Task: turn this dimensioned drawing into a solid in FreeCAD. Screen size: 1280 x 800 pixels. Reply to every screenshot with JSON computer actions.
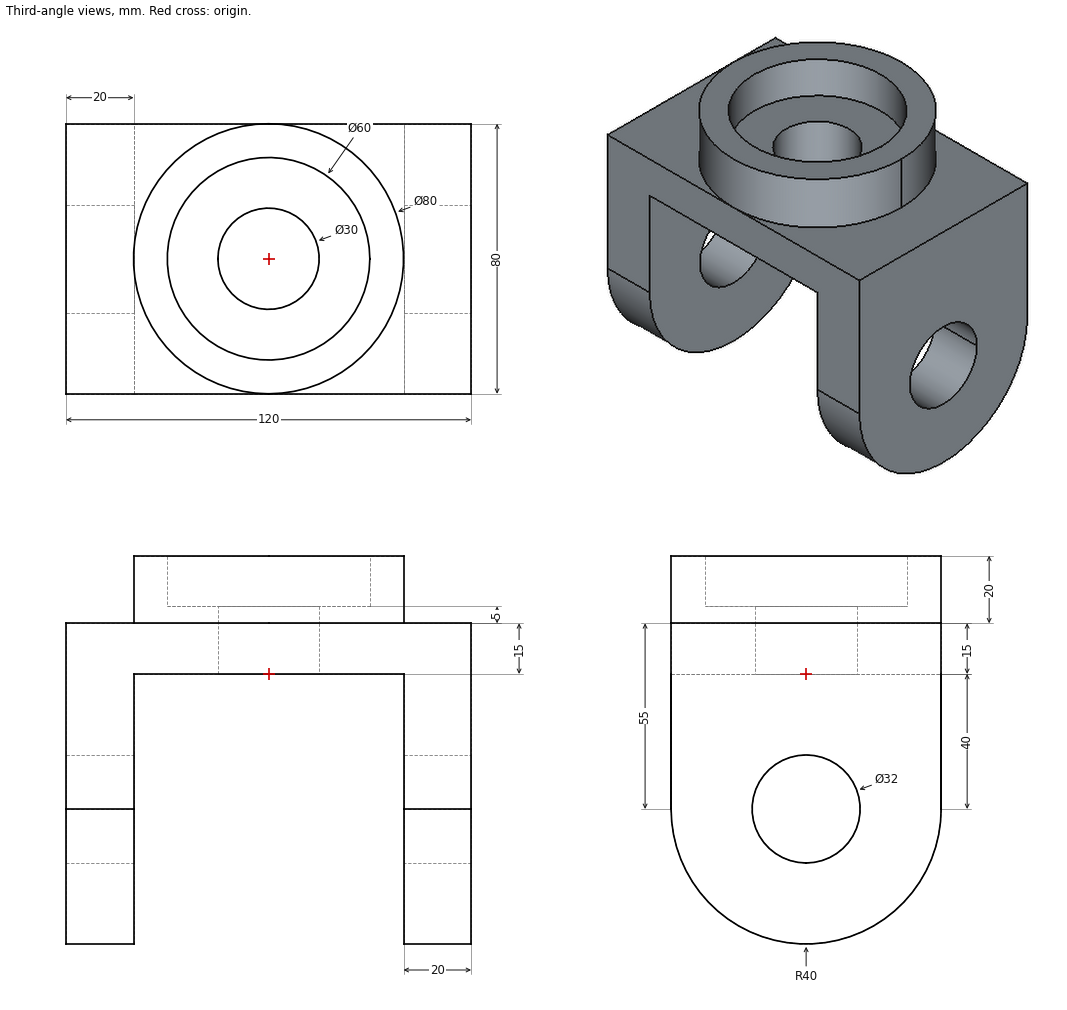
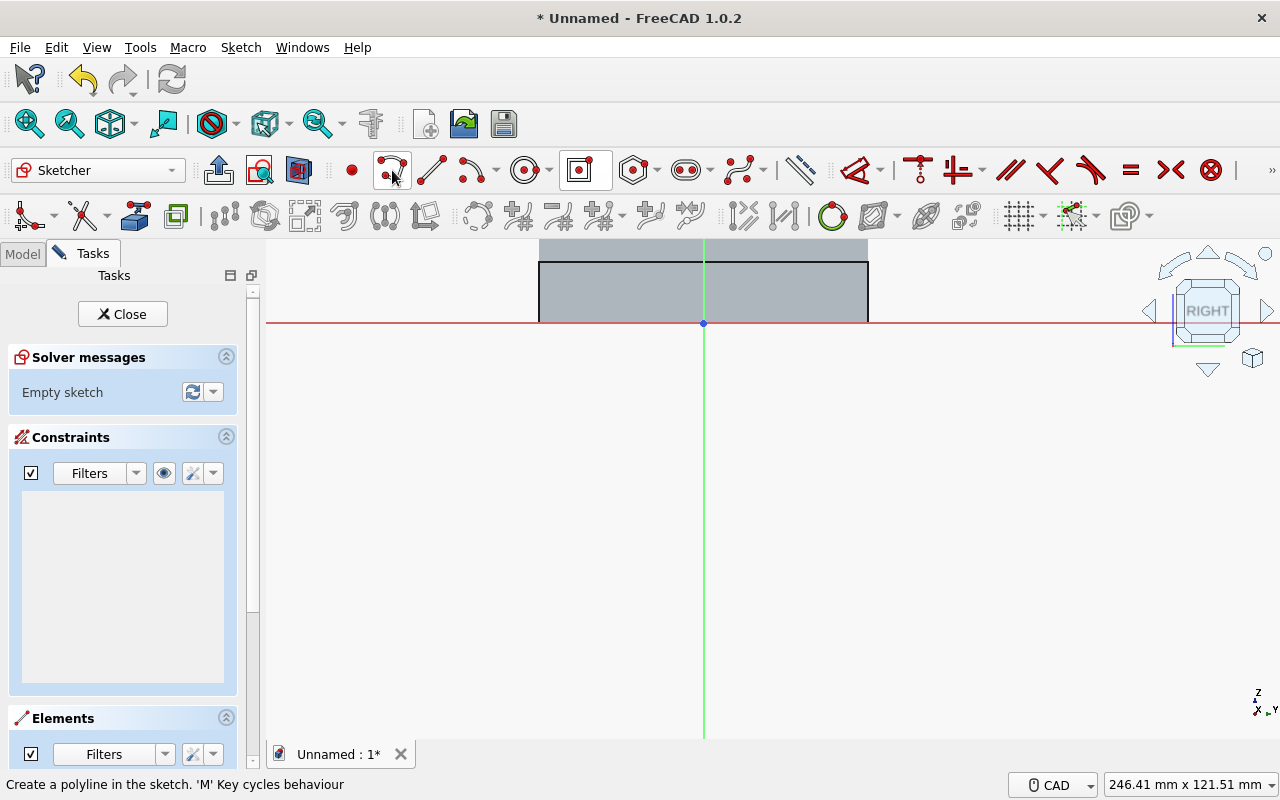
{"action": "left_click", "coordinate": [868, 488]}
{"action": "left_click", "coordinate": [868, 323]}
{"action": "left_click", "coordinate": [539, 332]}
{"action": "left_click", "coordinate": [539, 488]}
{"action": "right_click", "coordinate": [539, 488]}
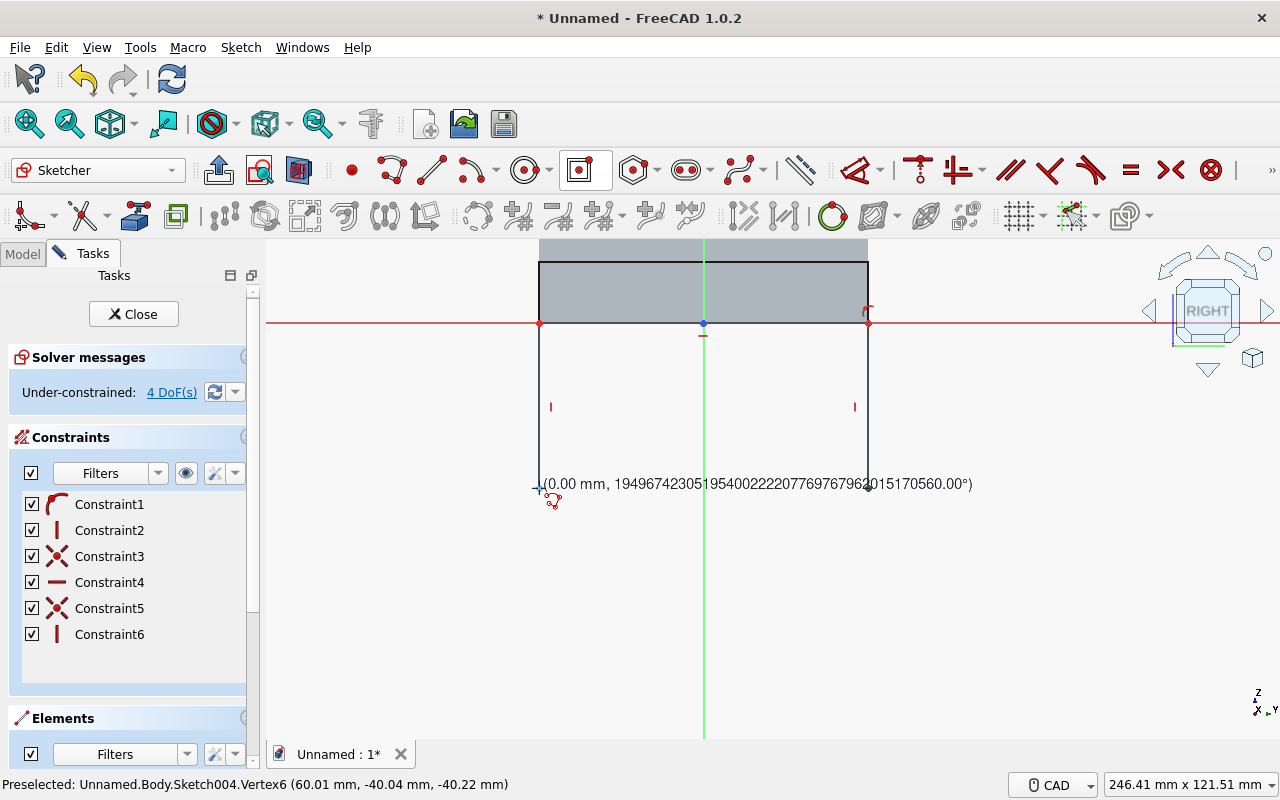
{"action": "key", "text": "g 3 a"}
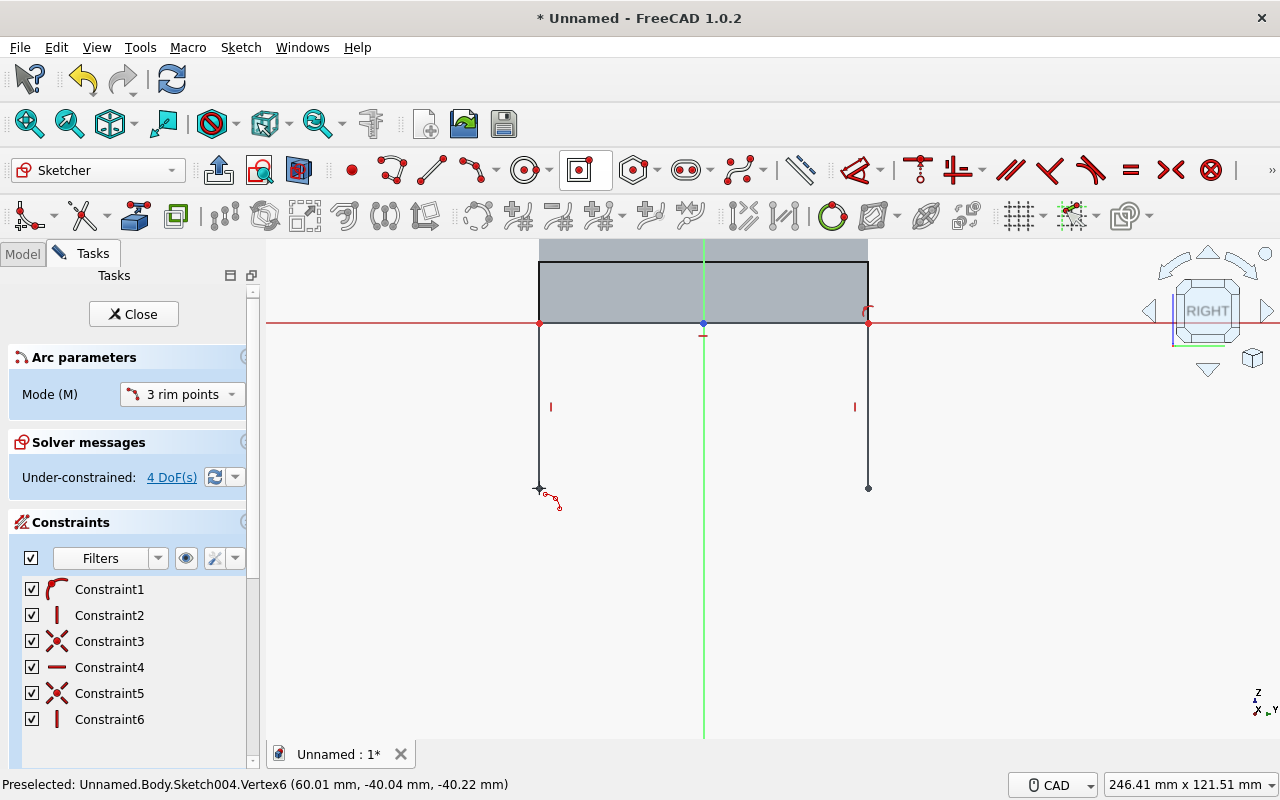
{"action": "left_click", "coordinate": [539, 489]}
{"action": "left_click", "coordinate": [868, 489]}
{"action": "left_click", "coordinate": [653, 645]}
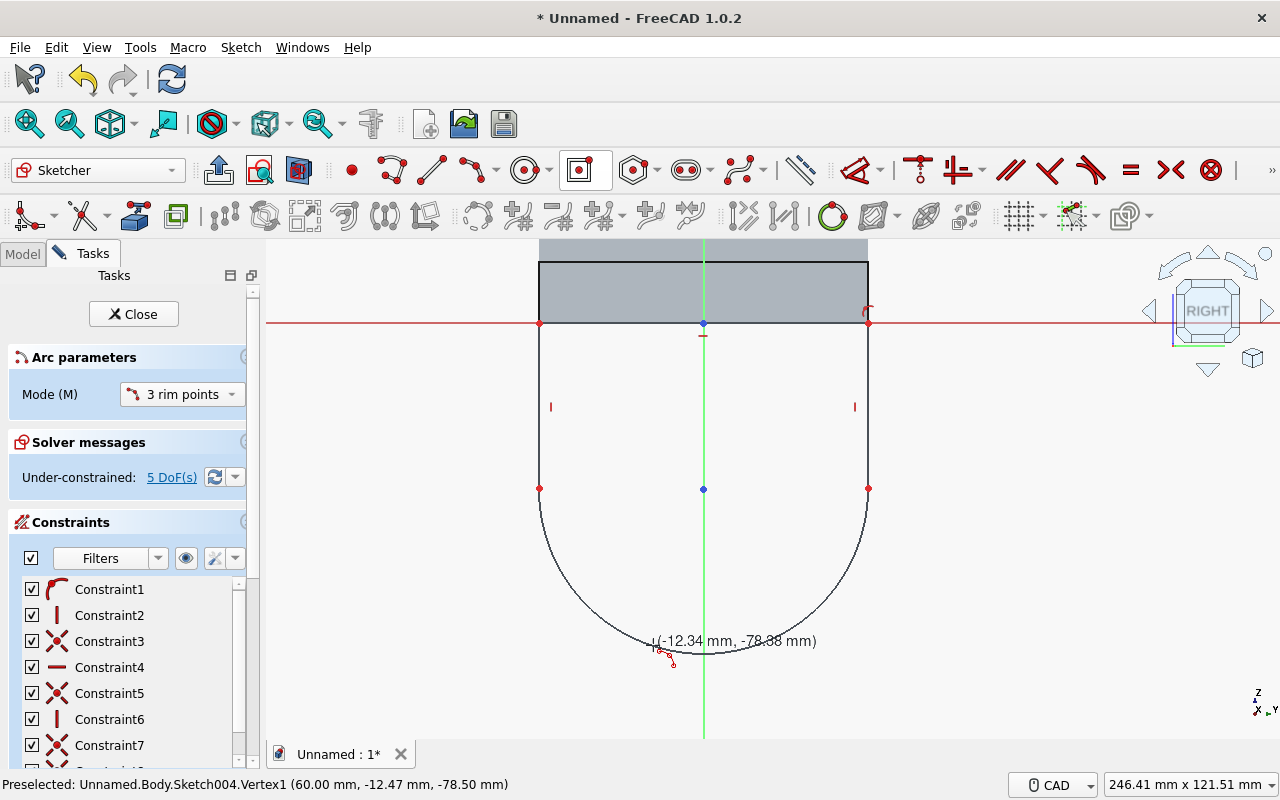
{"action": "left_click", "coordinate": [526, 170]}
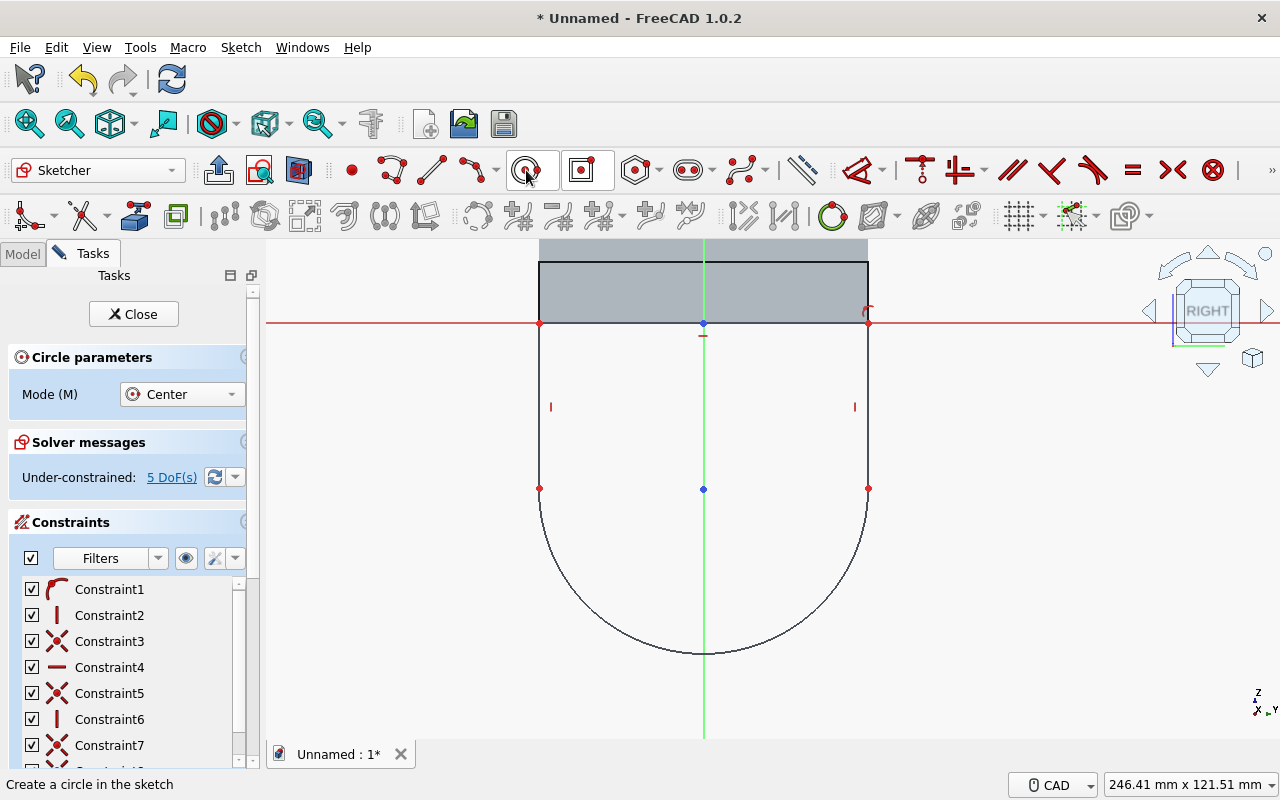
{"action": "left_click", "coordinate": [704, 488]}
{"action": "left_click", "coordinate": [750, 442]}
{"action": "key", "text": "Escape"}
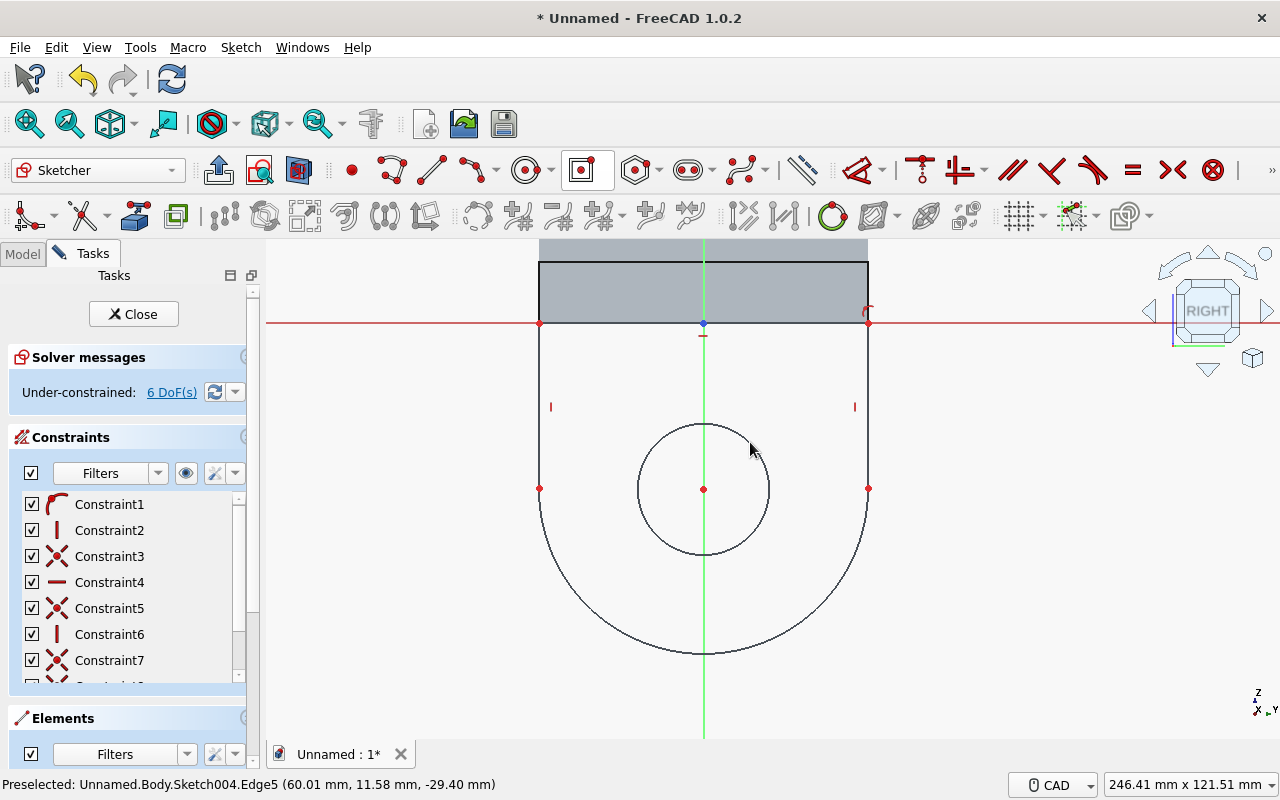
{"action": "left_click", "coordinate": [704, 489]}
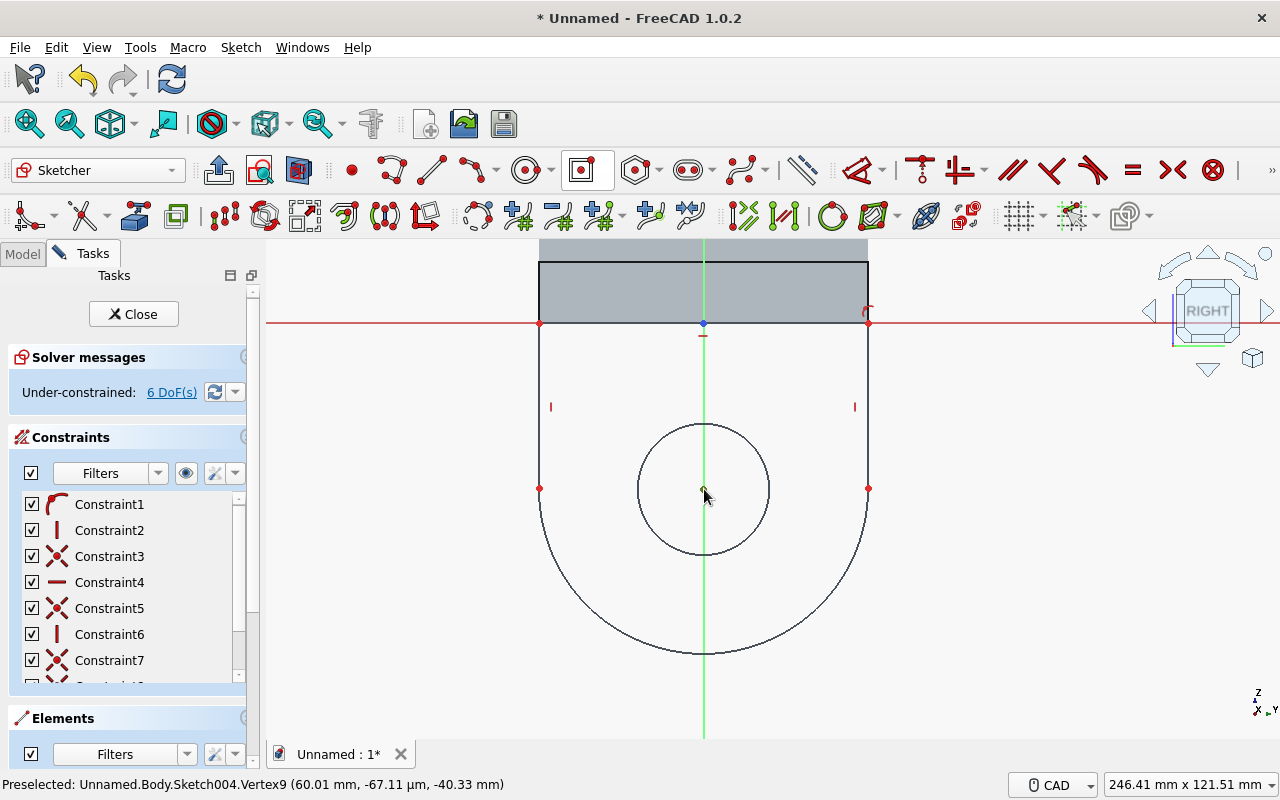
{"action": "left_click", "coordinate": [704, 616]}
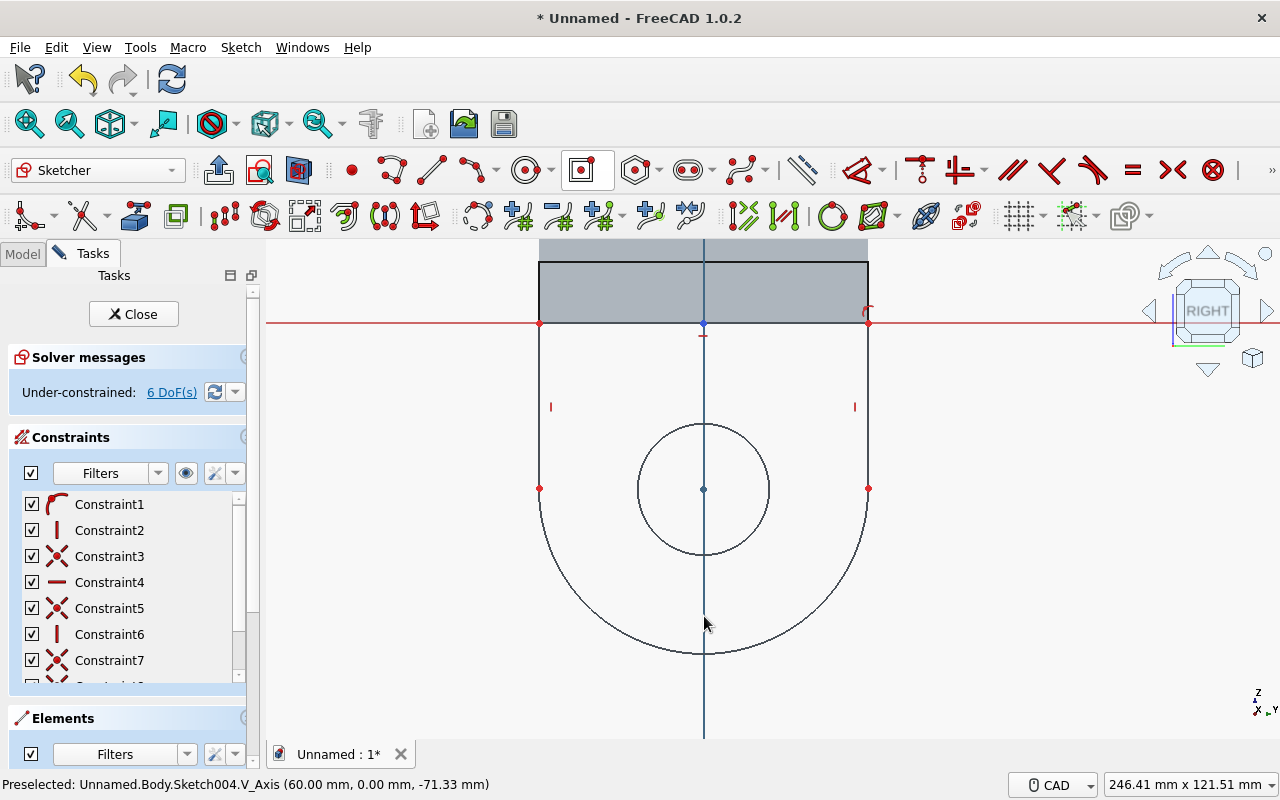
{"action": "left_click", "coordinate": [920, 170]}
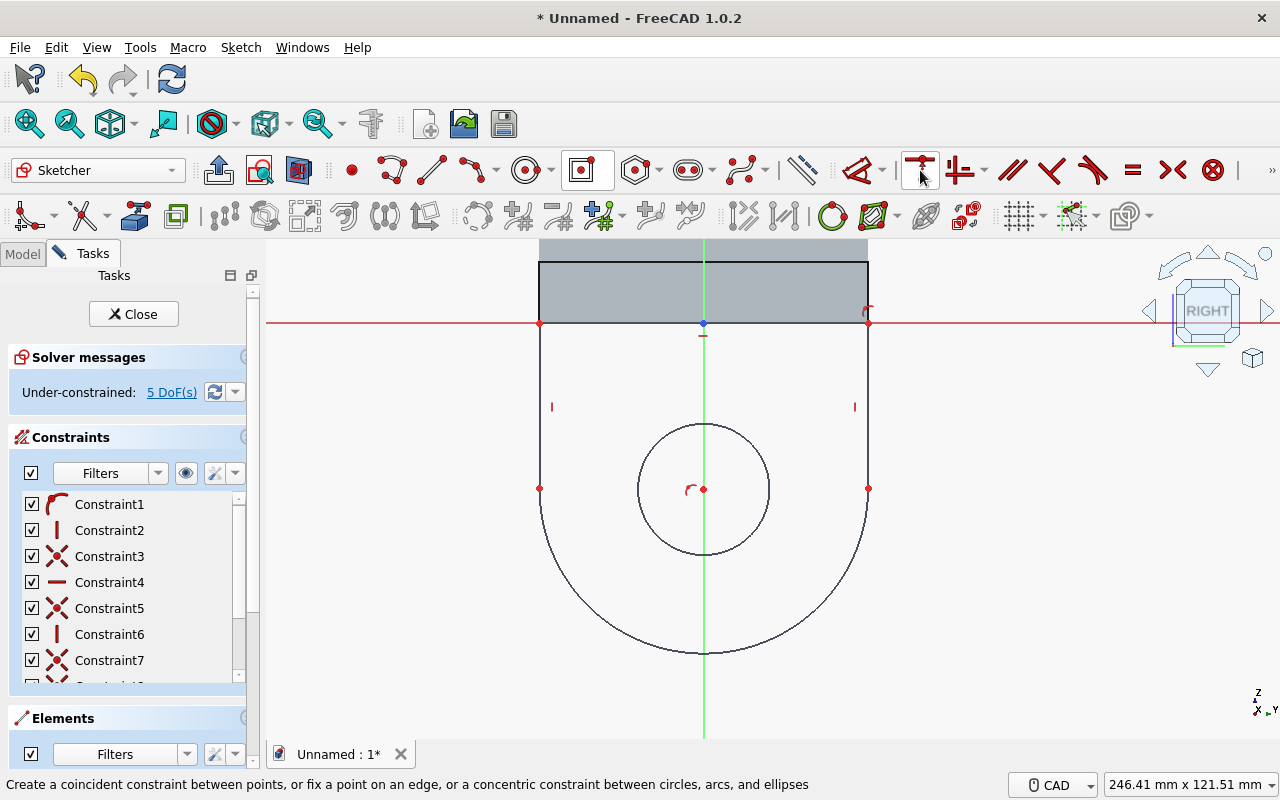
{"action": "key", "text": "d"}